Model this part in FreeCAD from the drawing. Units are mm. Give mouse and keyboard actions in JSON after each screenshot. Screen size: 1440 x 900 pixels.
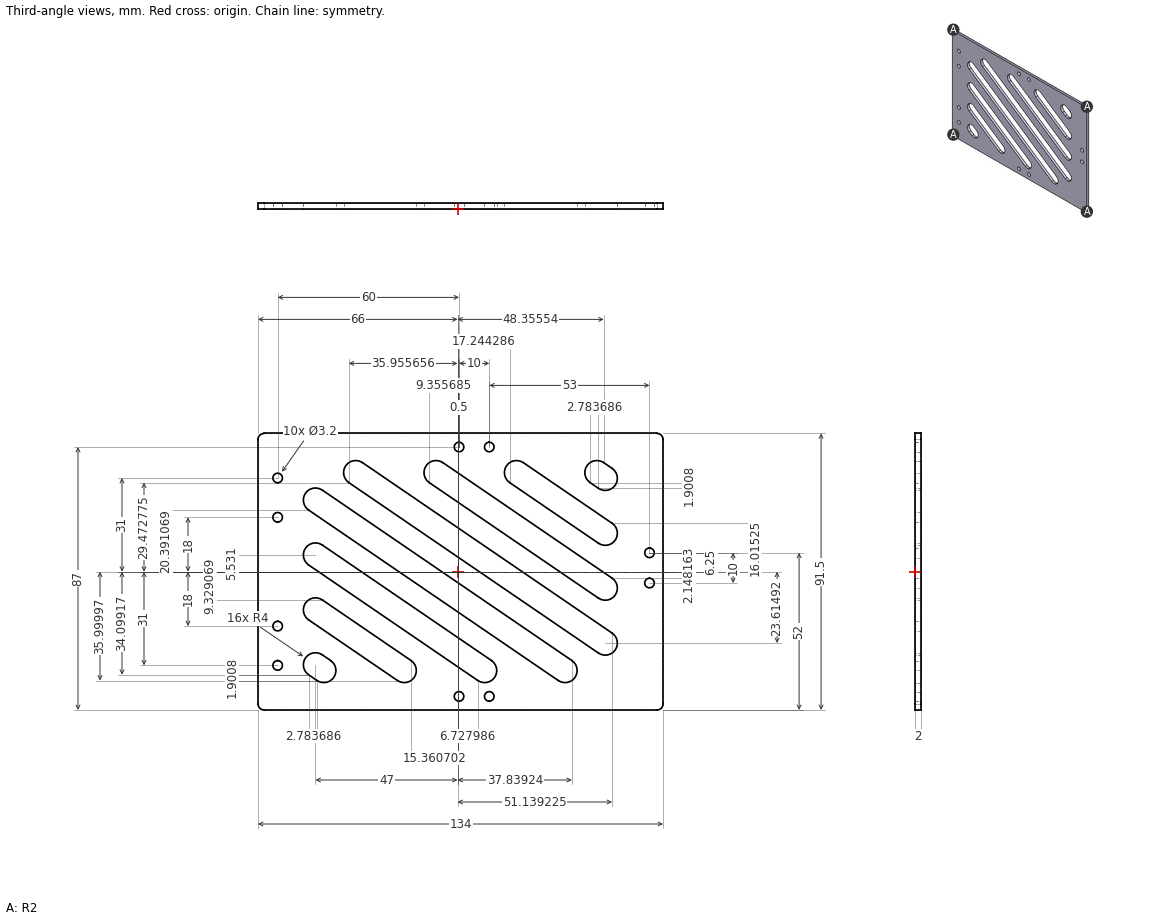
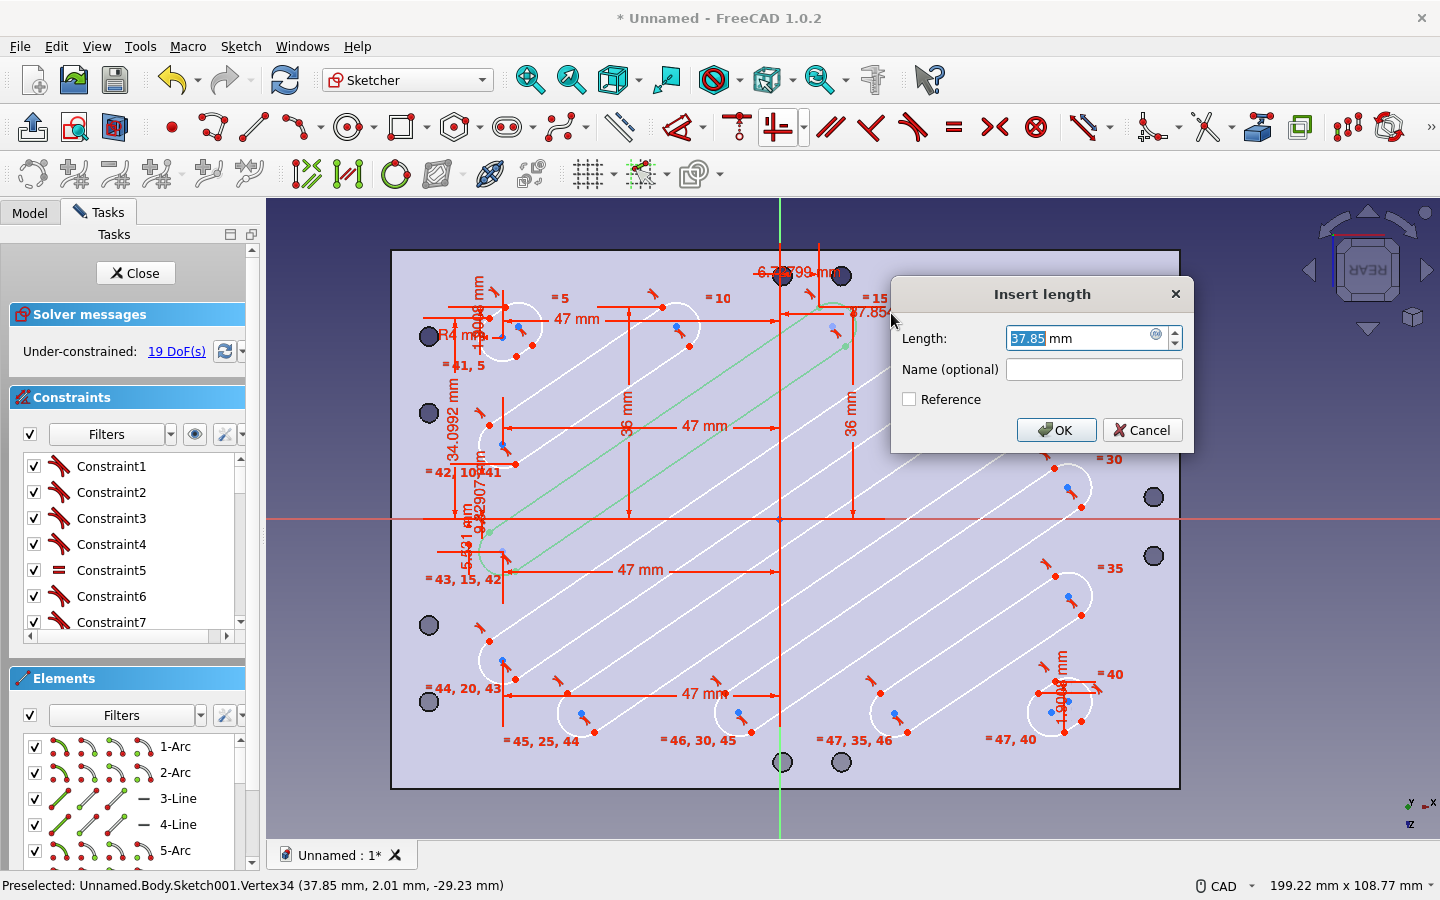
{"action": "type", "text": "37.83924"}
{"action": "key", "text": "Return"}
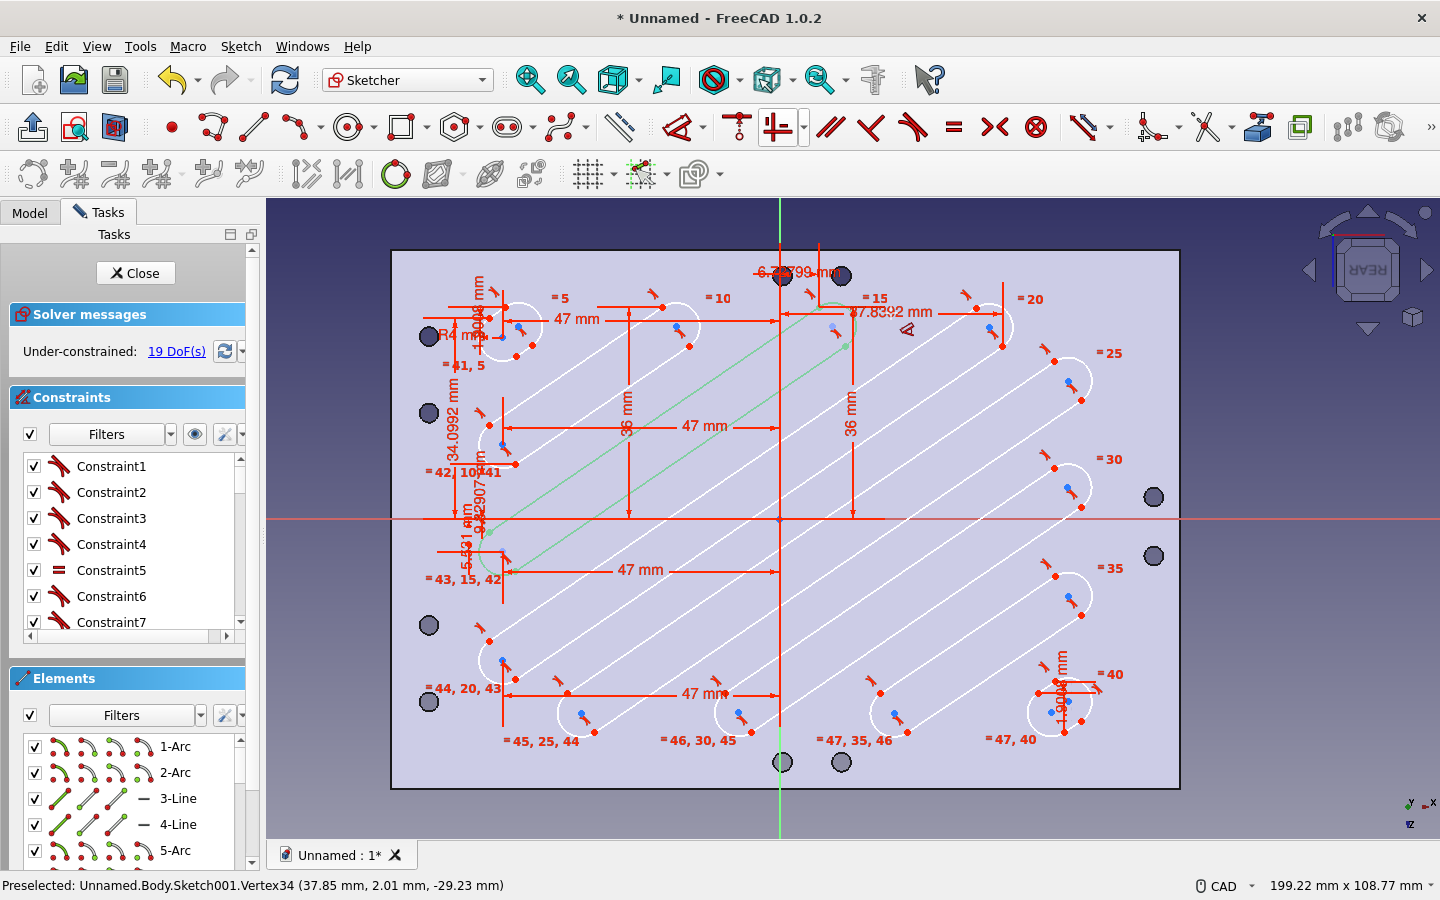
{"action": "left_click", "coordinate": [976, 308]}
{"action": "left_click", "coordinate": [1010, 414]}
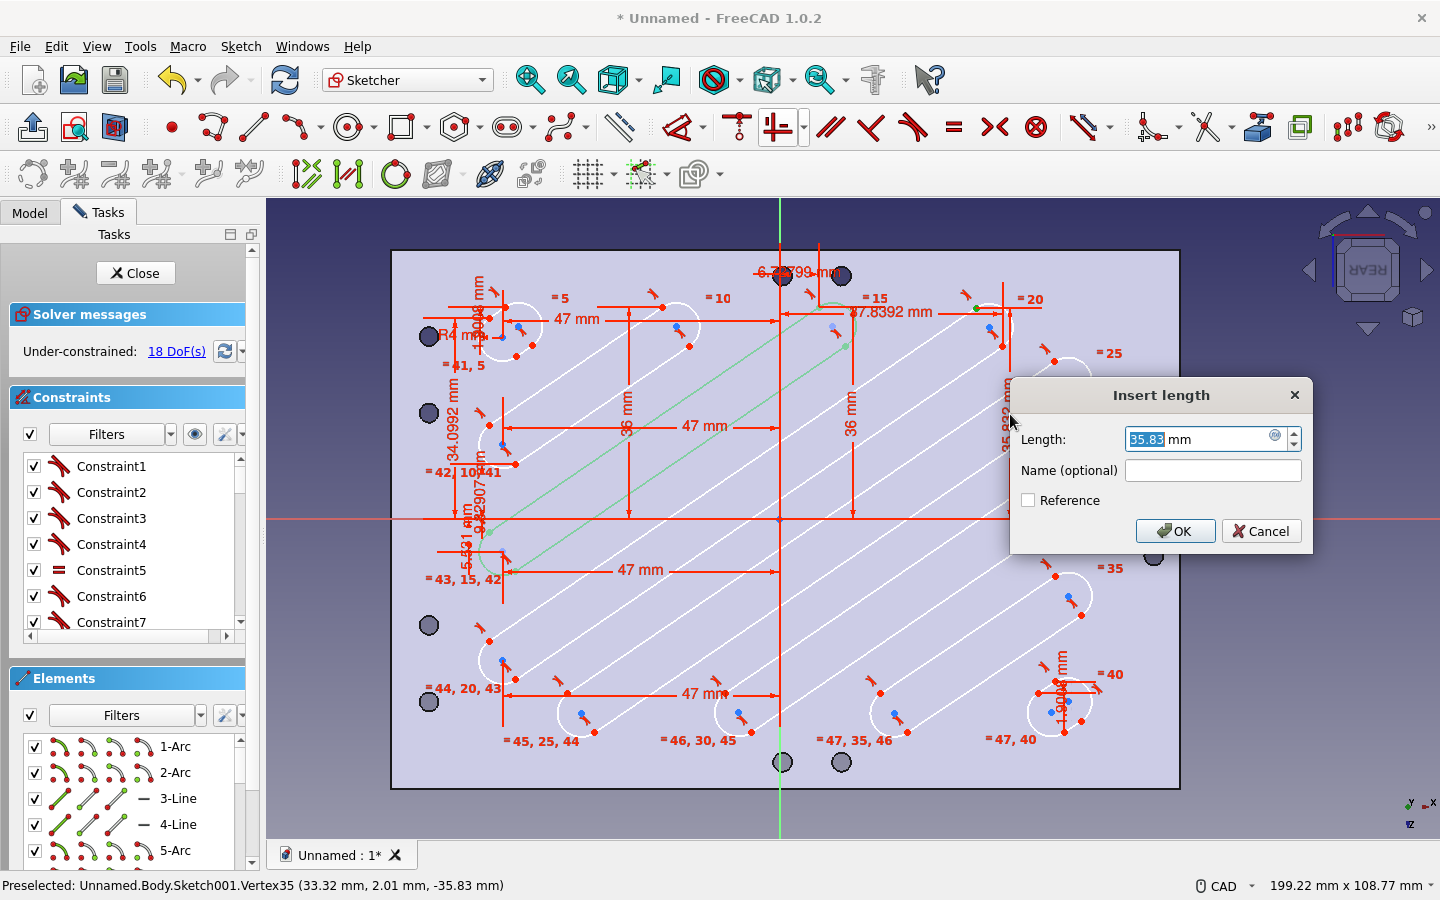
{"action": "type", "text": "35.99997"}
{"action": "key", "text": "Return"}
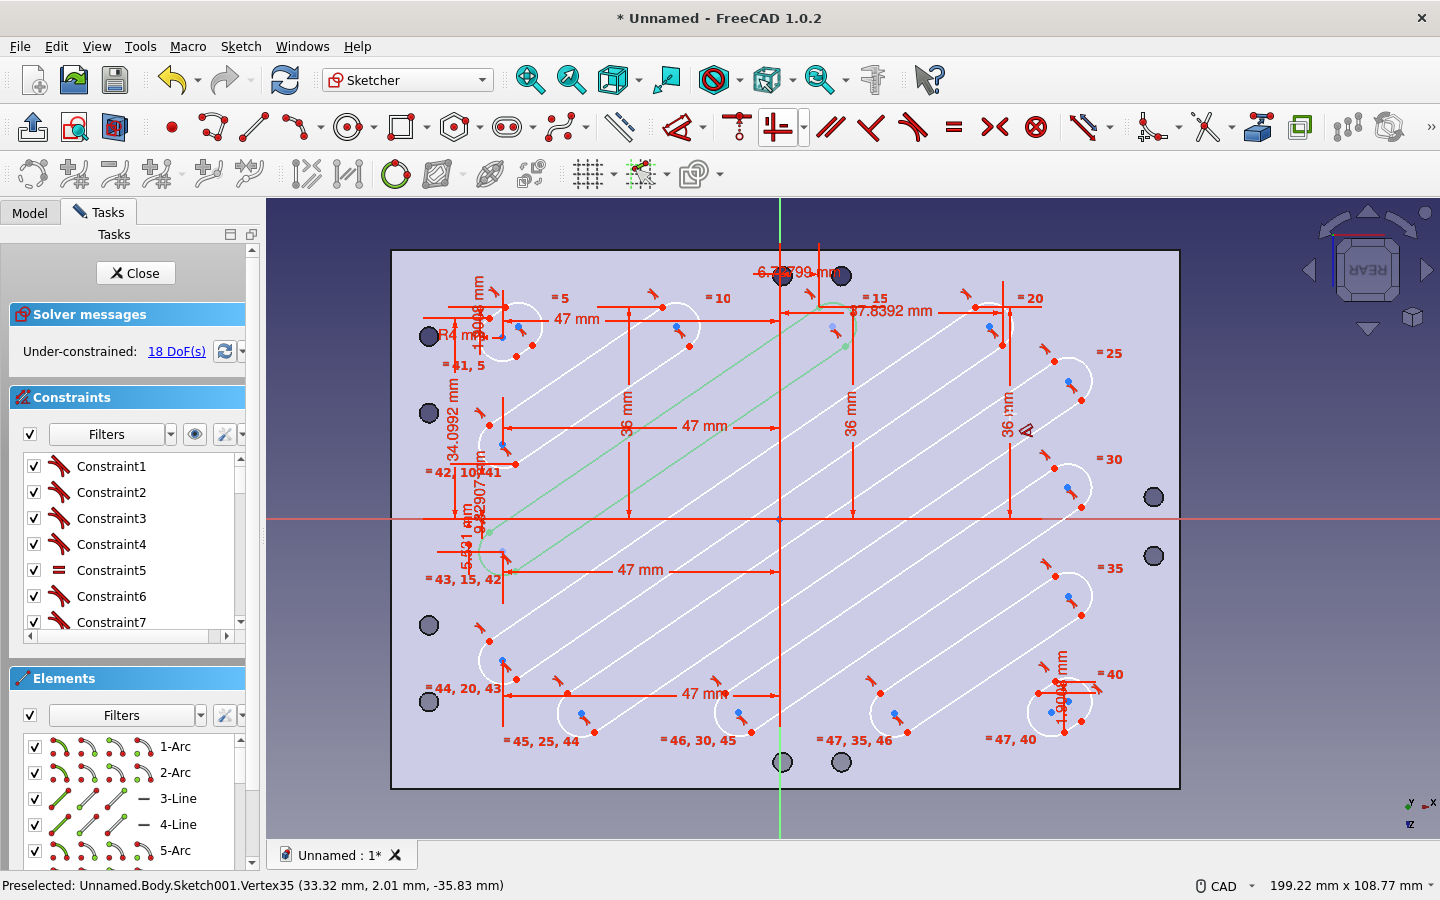
{"action": "left_click", "coordinate": [725, 693]}
{"action": "left_click", "coordinate": [752, 485]}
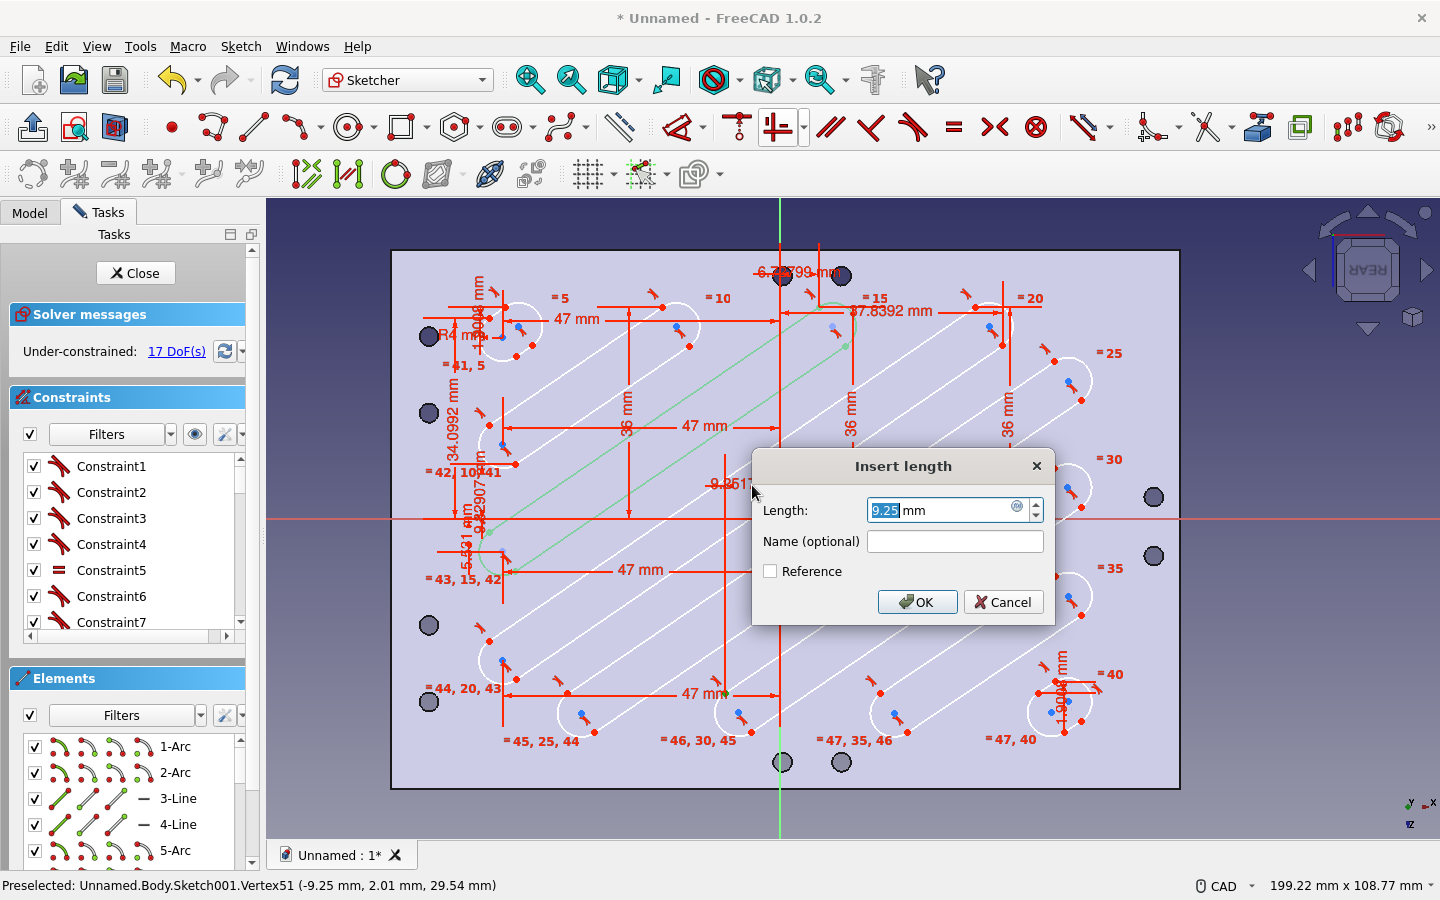
{"action": "type", "text": "9.355685"}
{"action": "key", "text": "Return"}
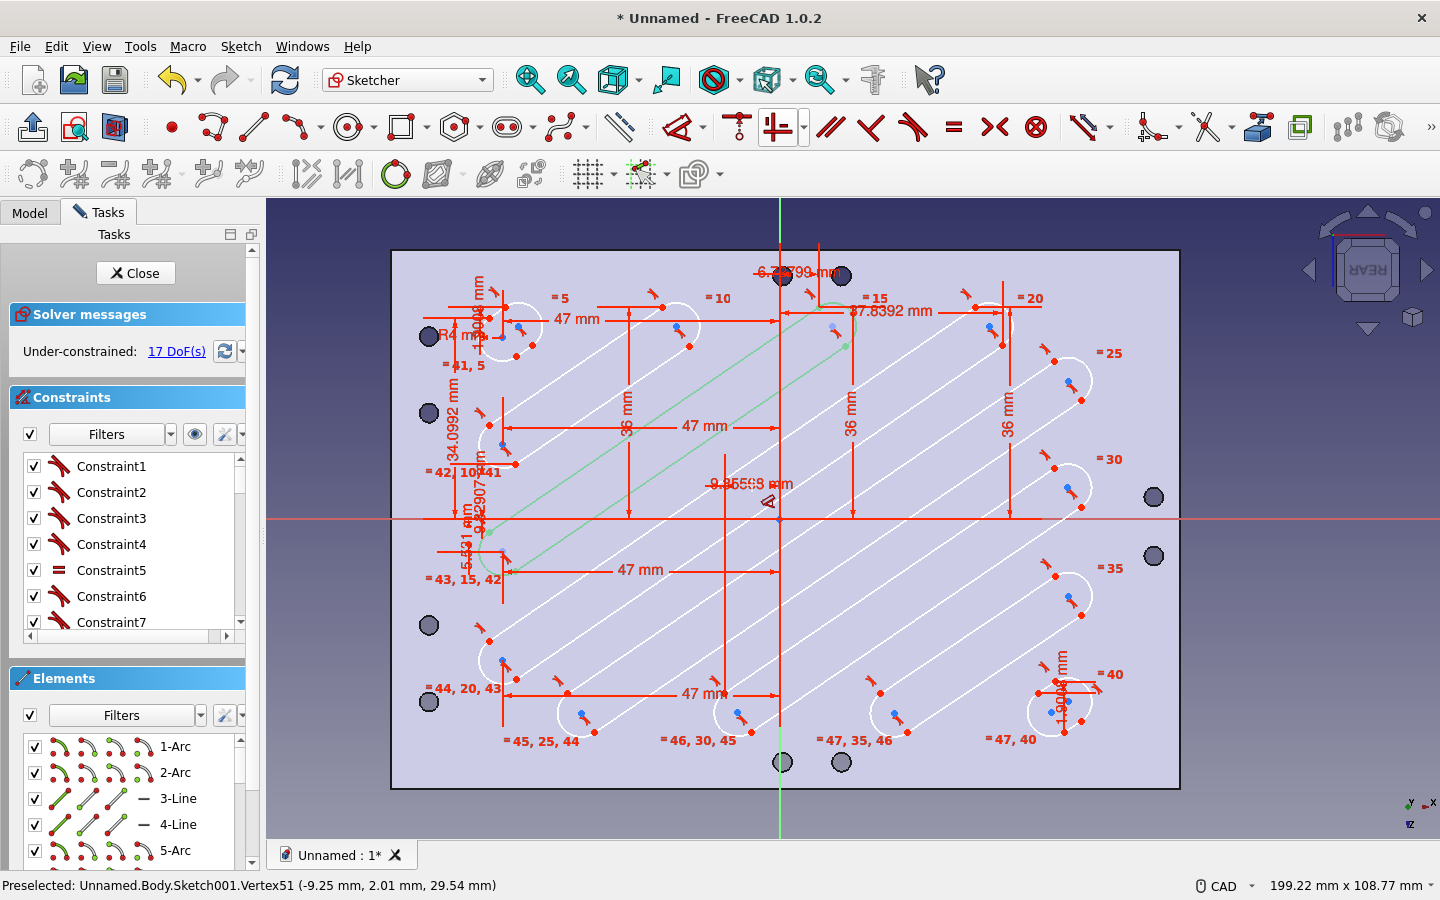
{"action": "scroll", "coordinate": [1081, 507], "scroll_direction": "up", "scroll_amount": 6}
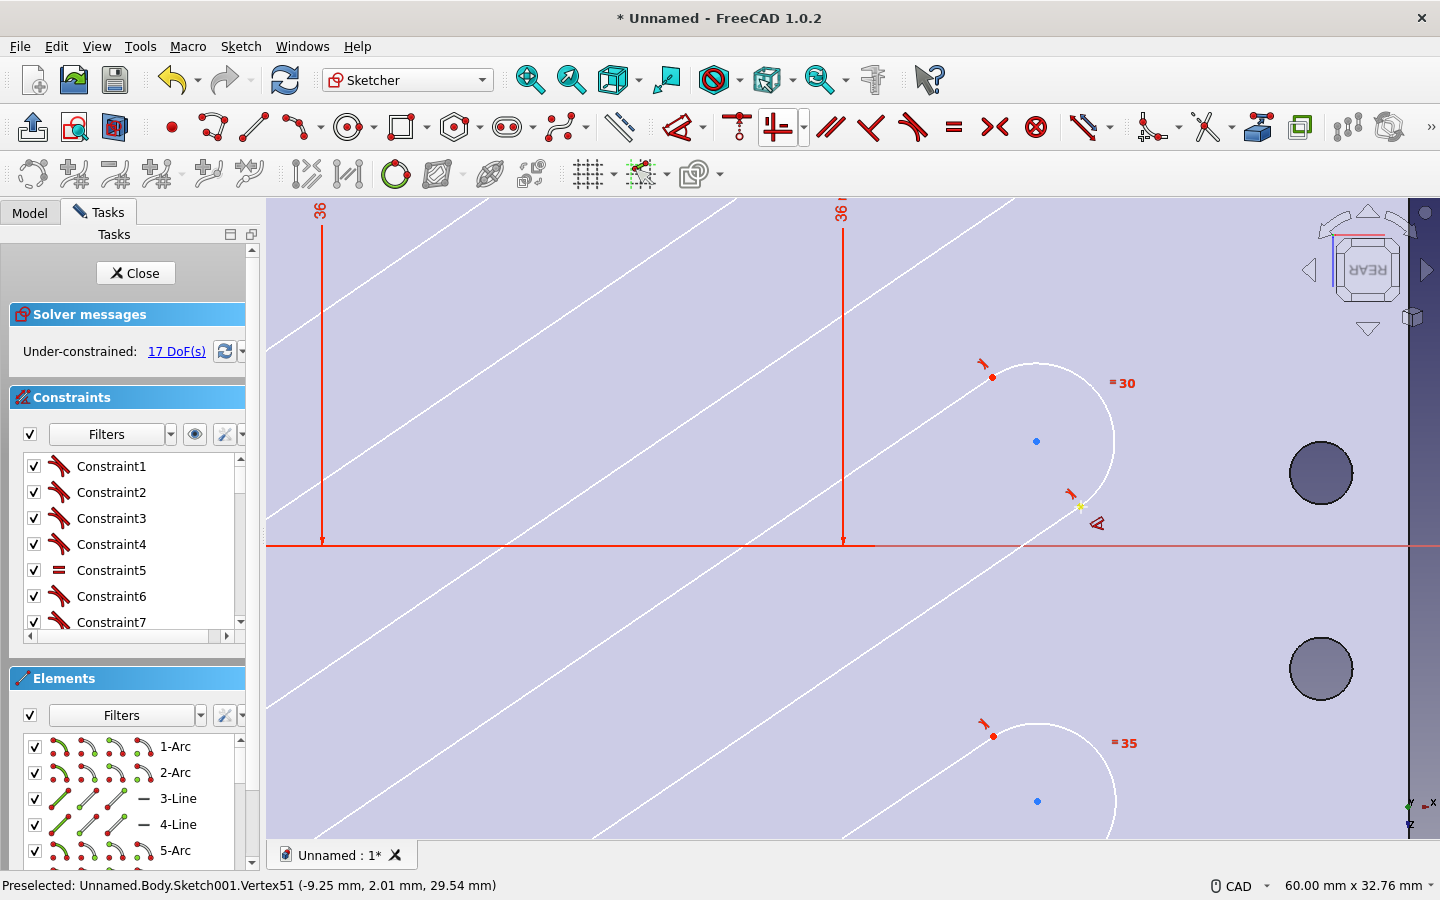
{"action": "left_click", "coordinate": [1080, 506]}
{"action": "left_click", "coordinate": [1114, 526]}